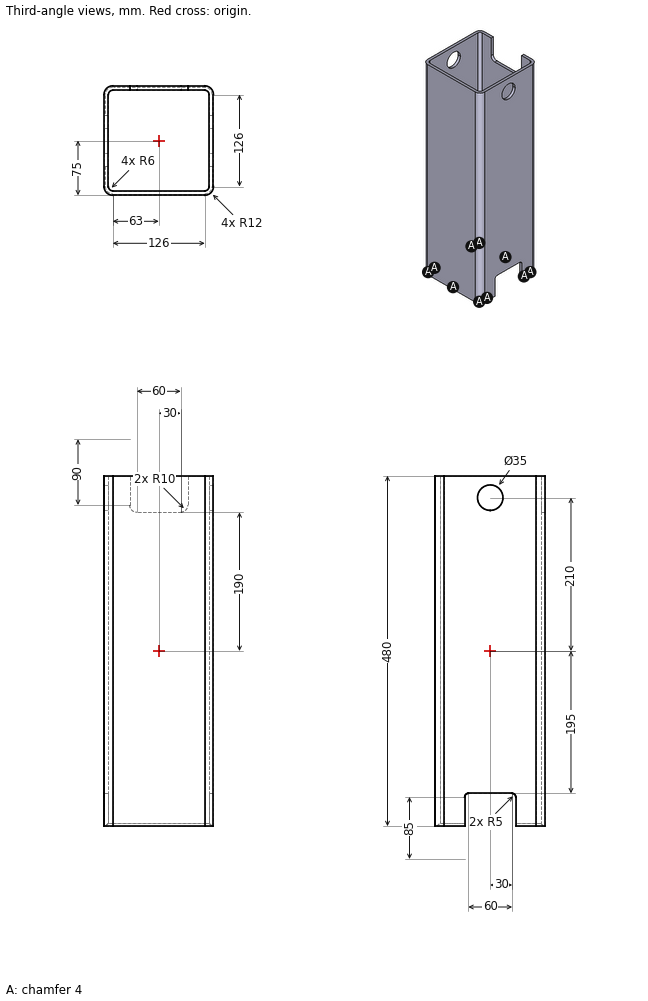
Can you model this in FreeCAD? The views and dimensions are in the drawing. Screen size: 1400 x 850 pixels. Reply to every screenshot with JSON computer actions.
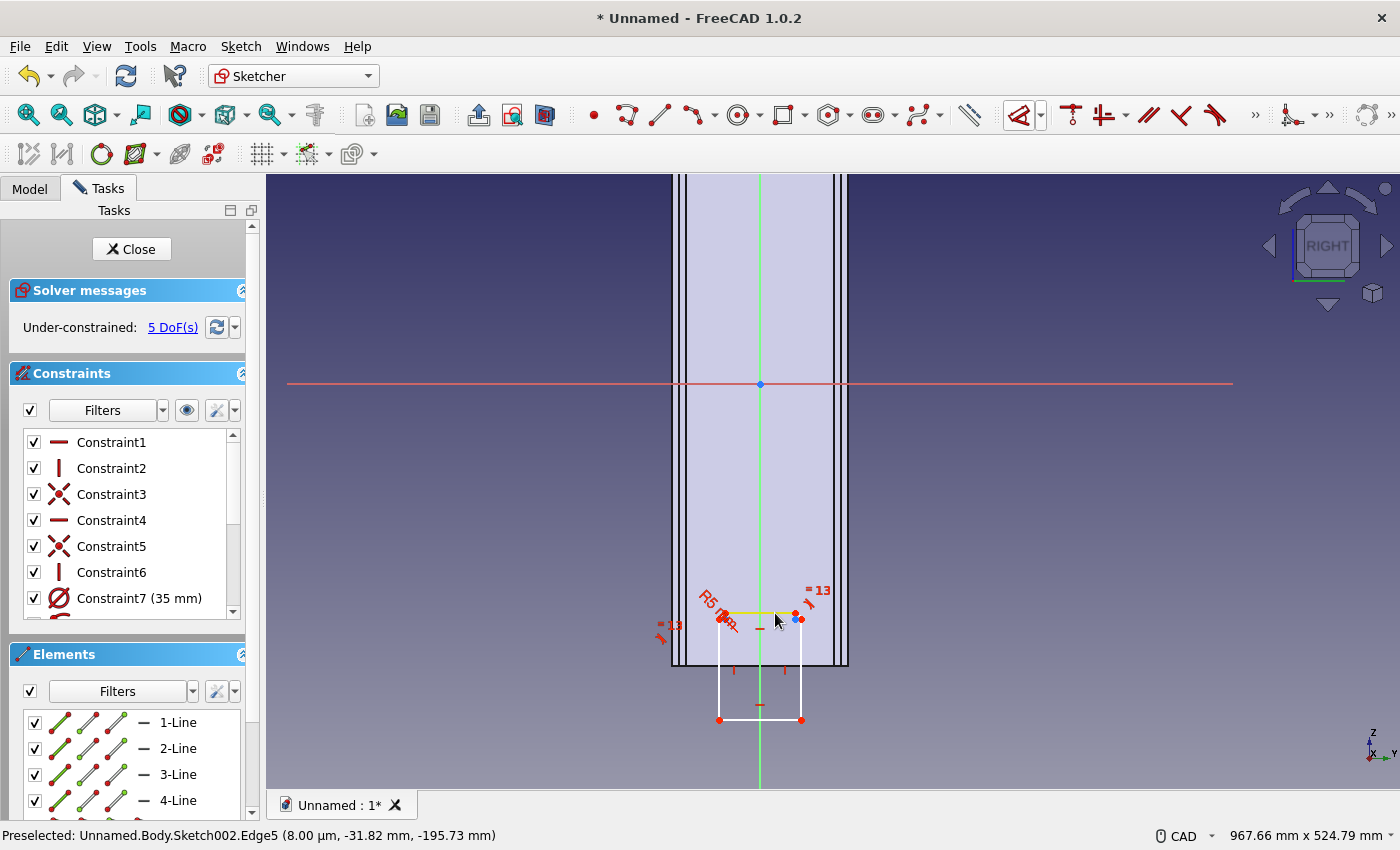
{"action": "left_click", "coordinate": [774, 613]}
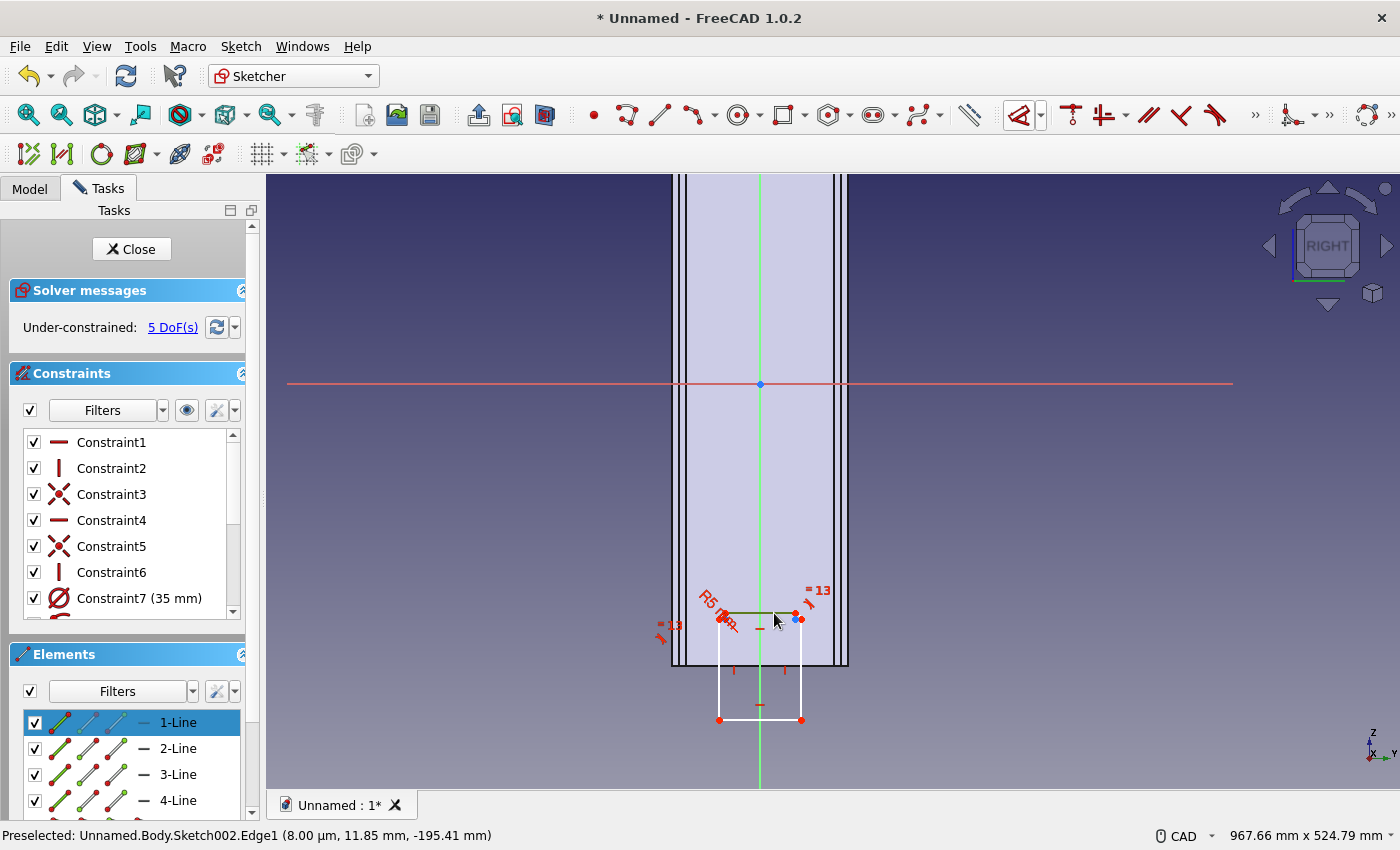
{"action": "key", "text": "l"}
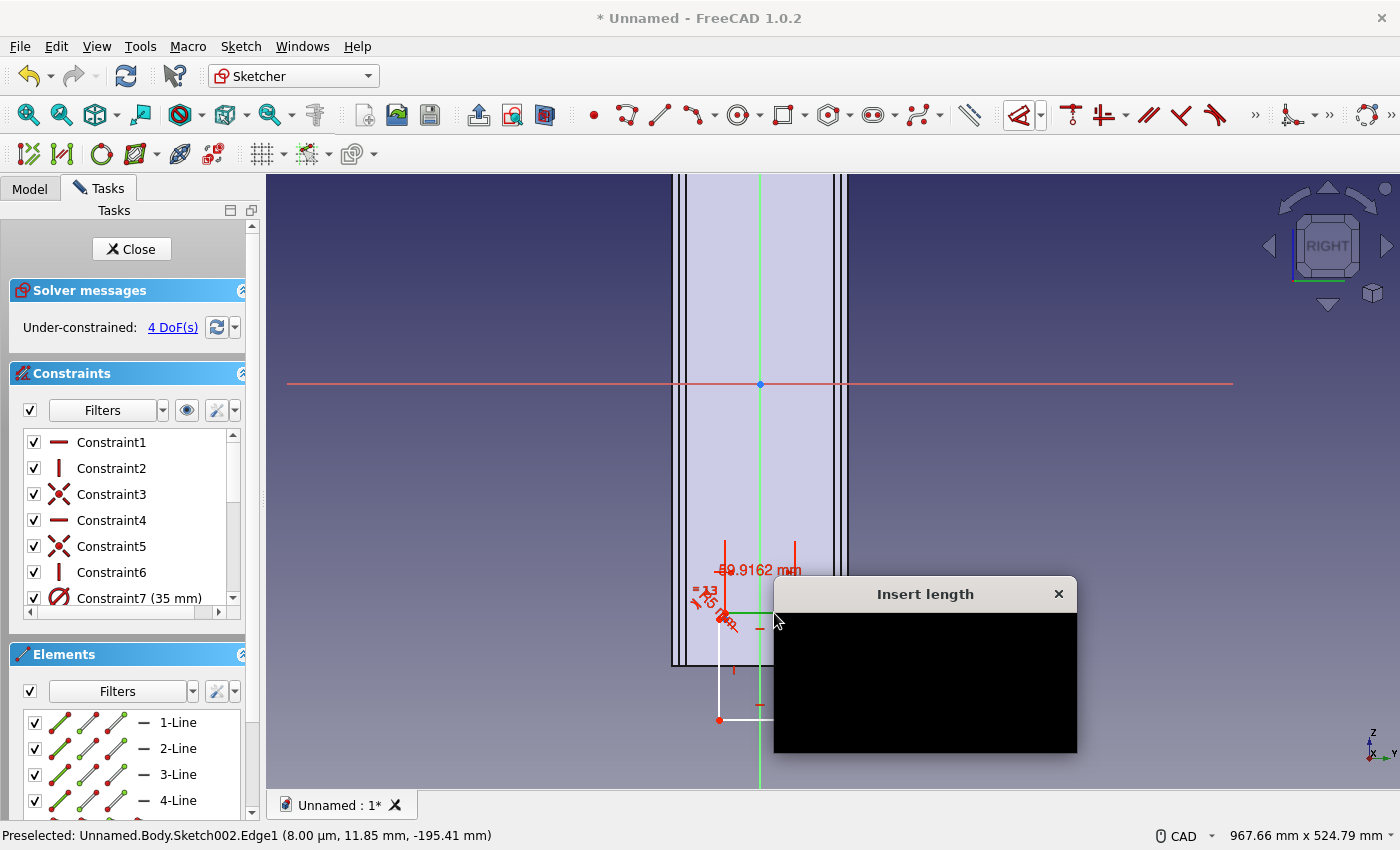
{"action": "type", "text": "60"}
{"action": "key", "text": "Return"}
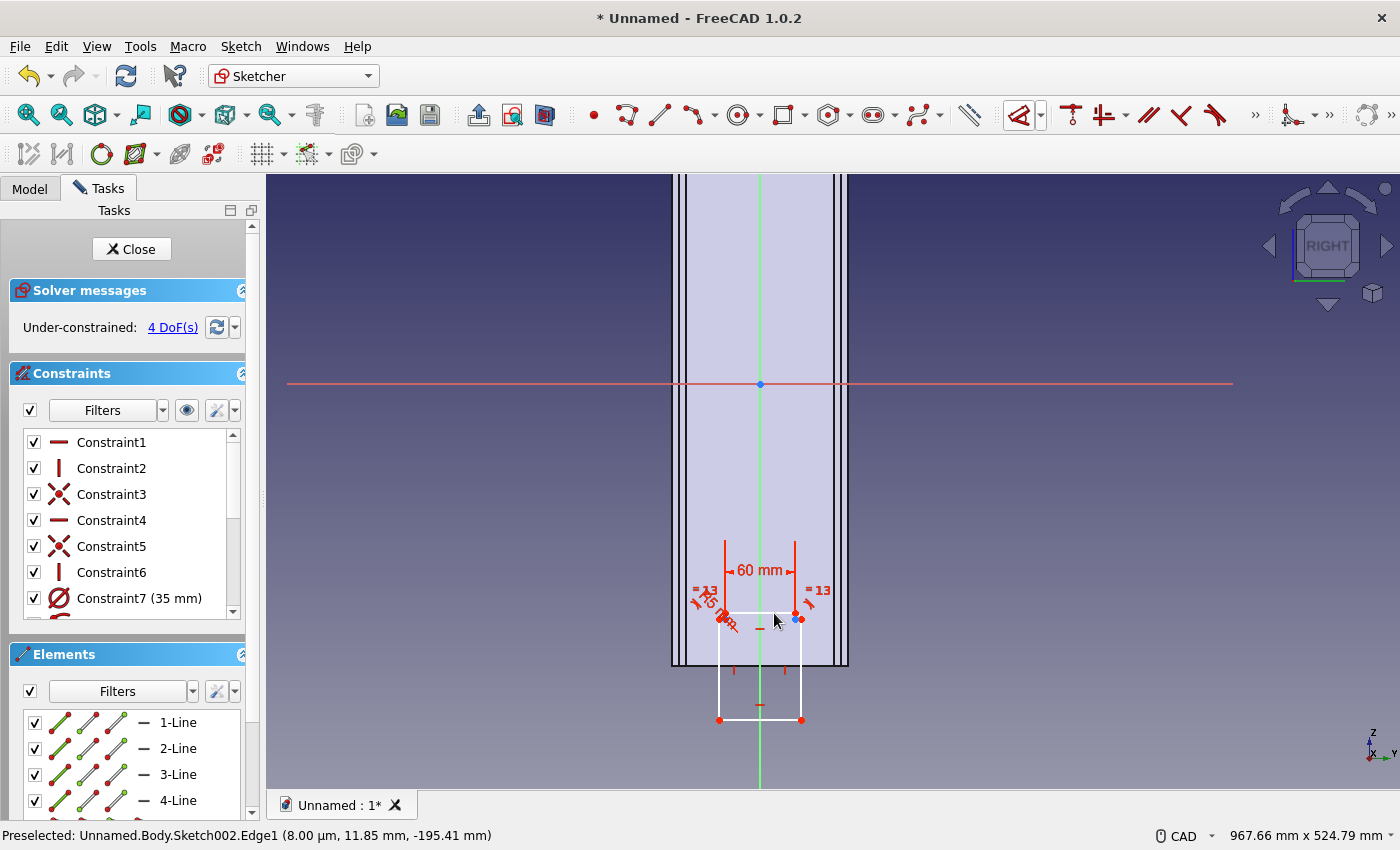
{"action": "left_click", "coordinate": [719, 650]}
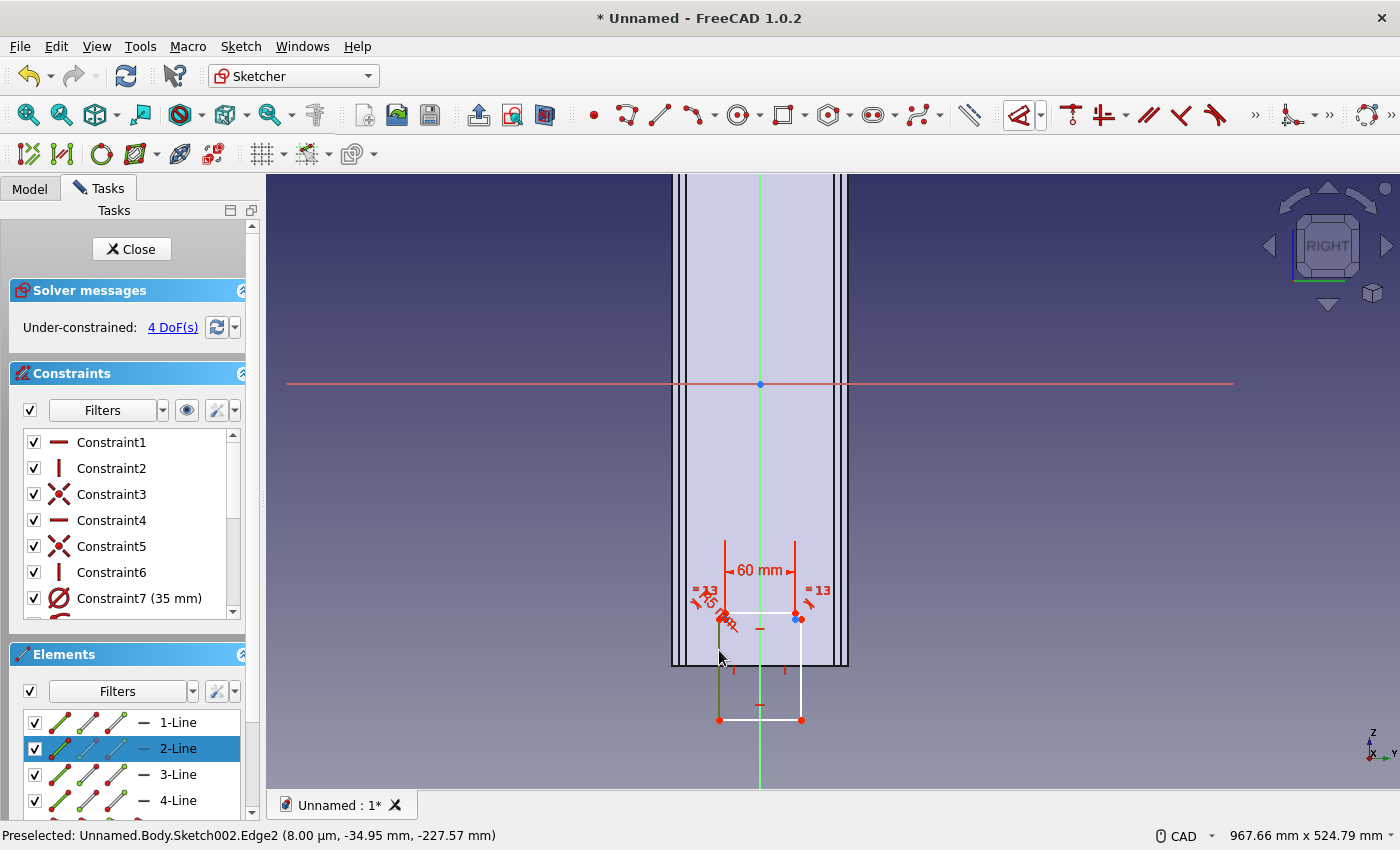
{"action": "key", "text": "i"}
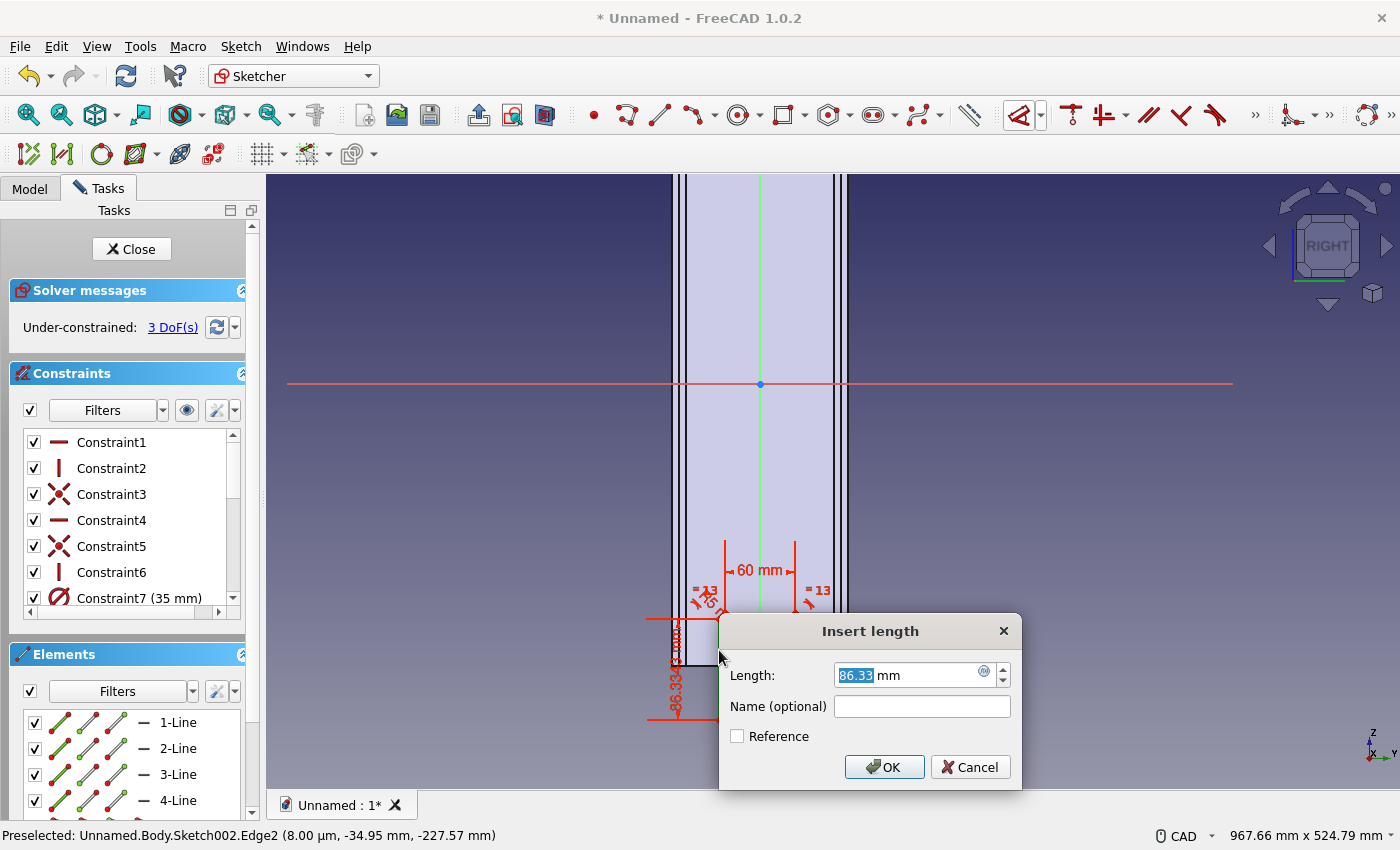
{"action": "type", "text": "85"}
{"action": "key", "text": "Return"}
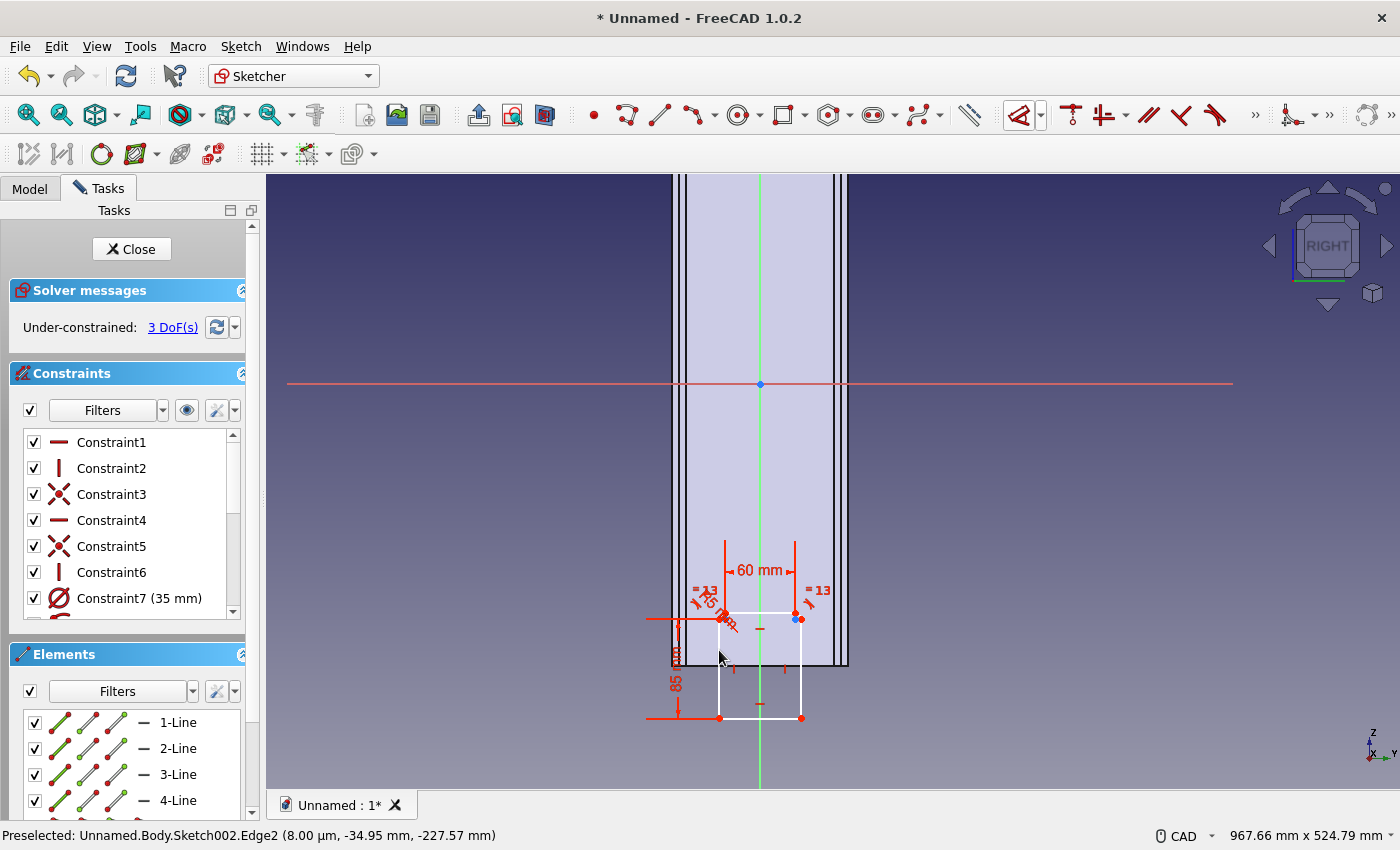
{"action": "scroll", "coordinate": [795, 613], "scroll_direction": "up", "scroll_amount": 4}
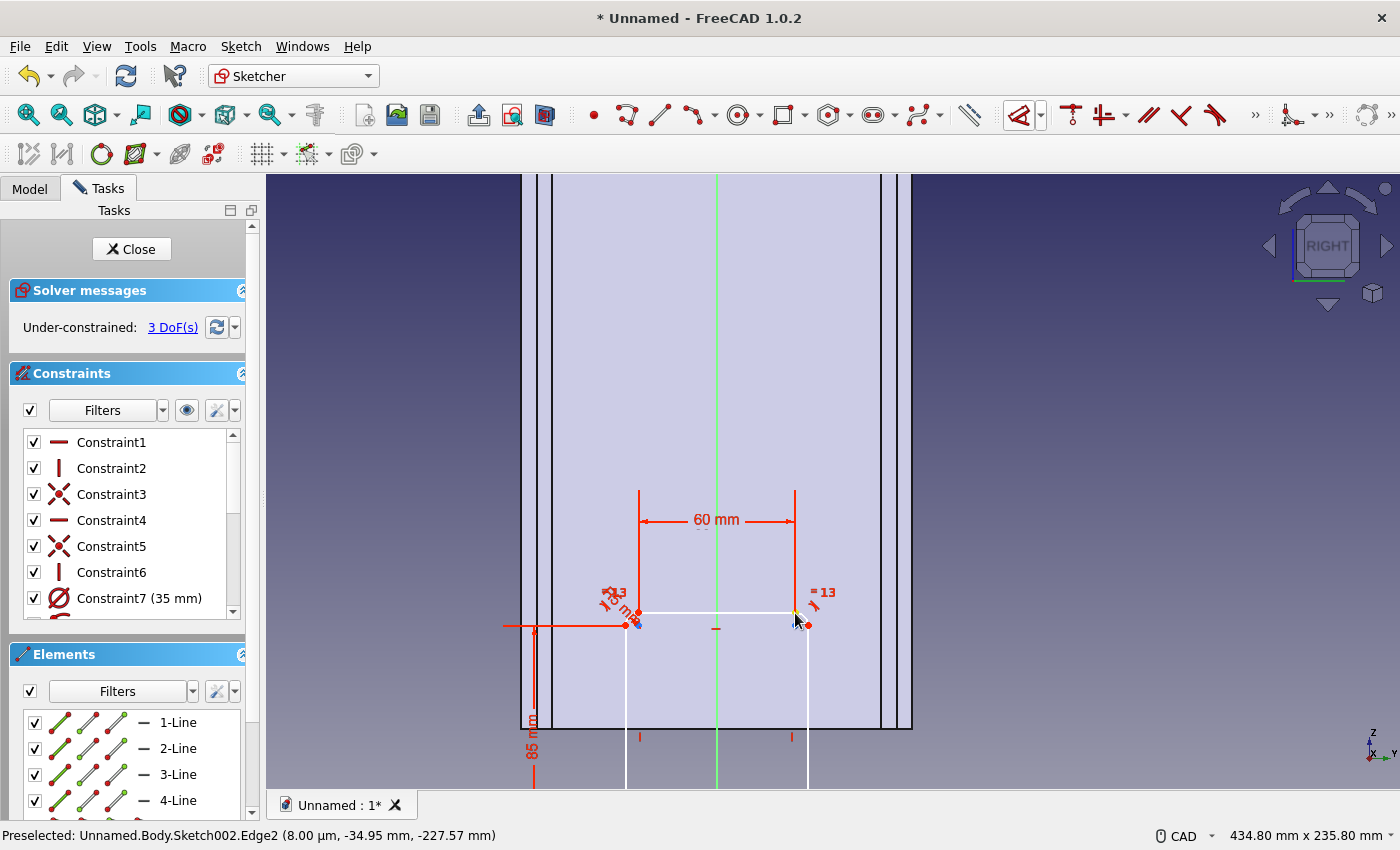
{"action": "left_click", "coordinate": [795, 613]}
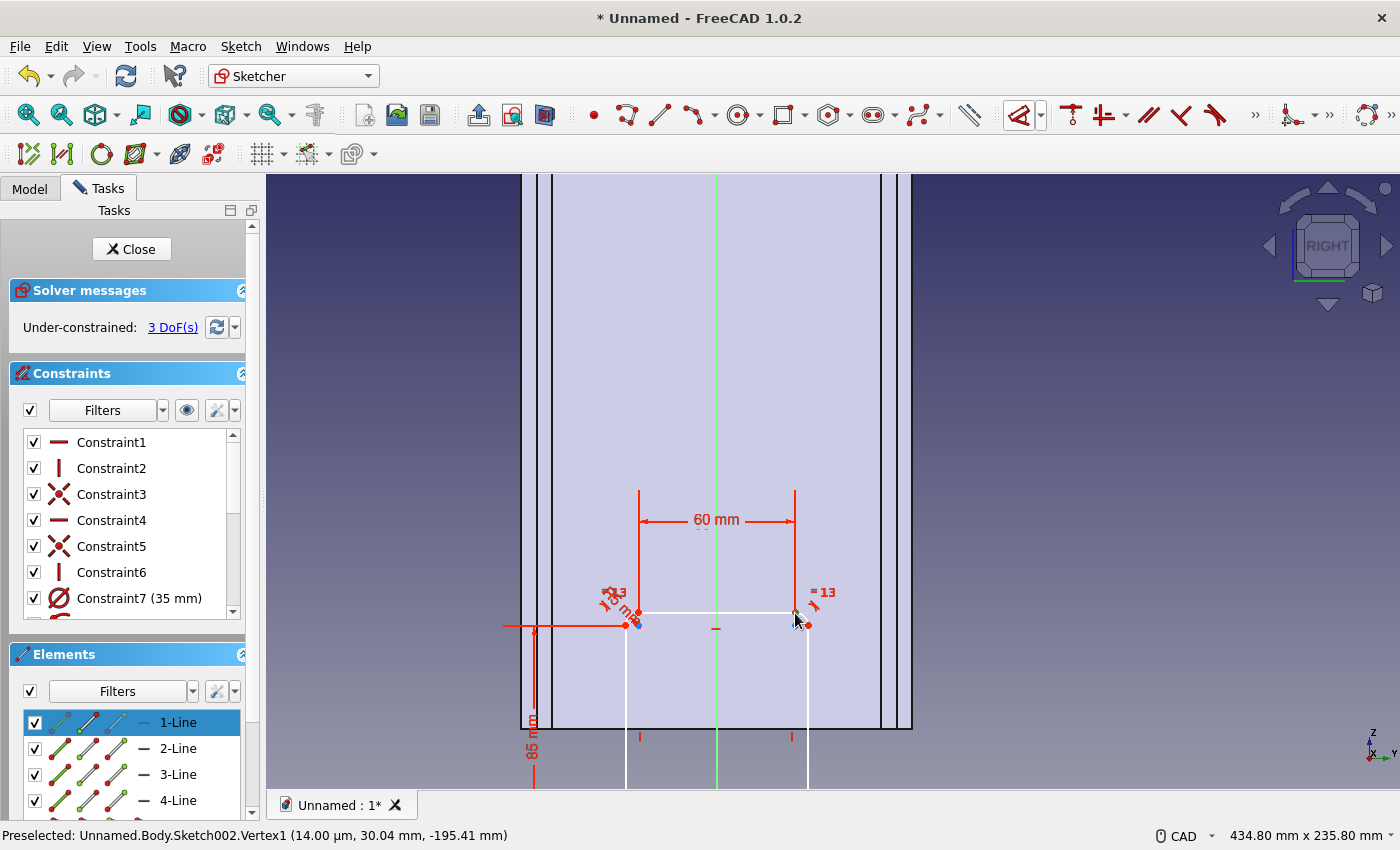
{"action": "key", "text": "l"}